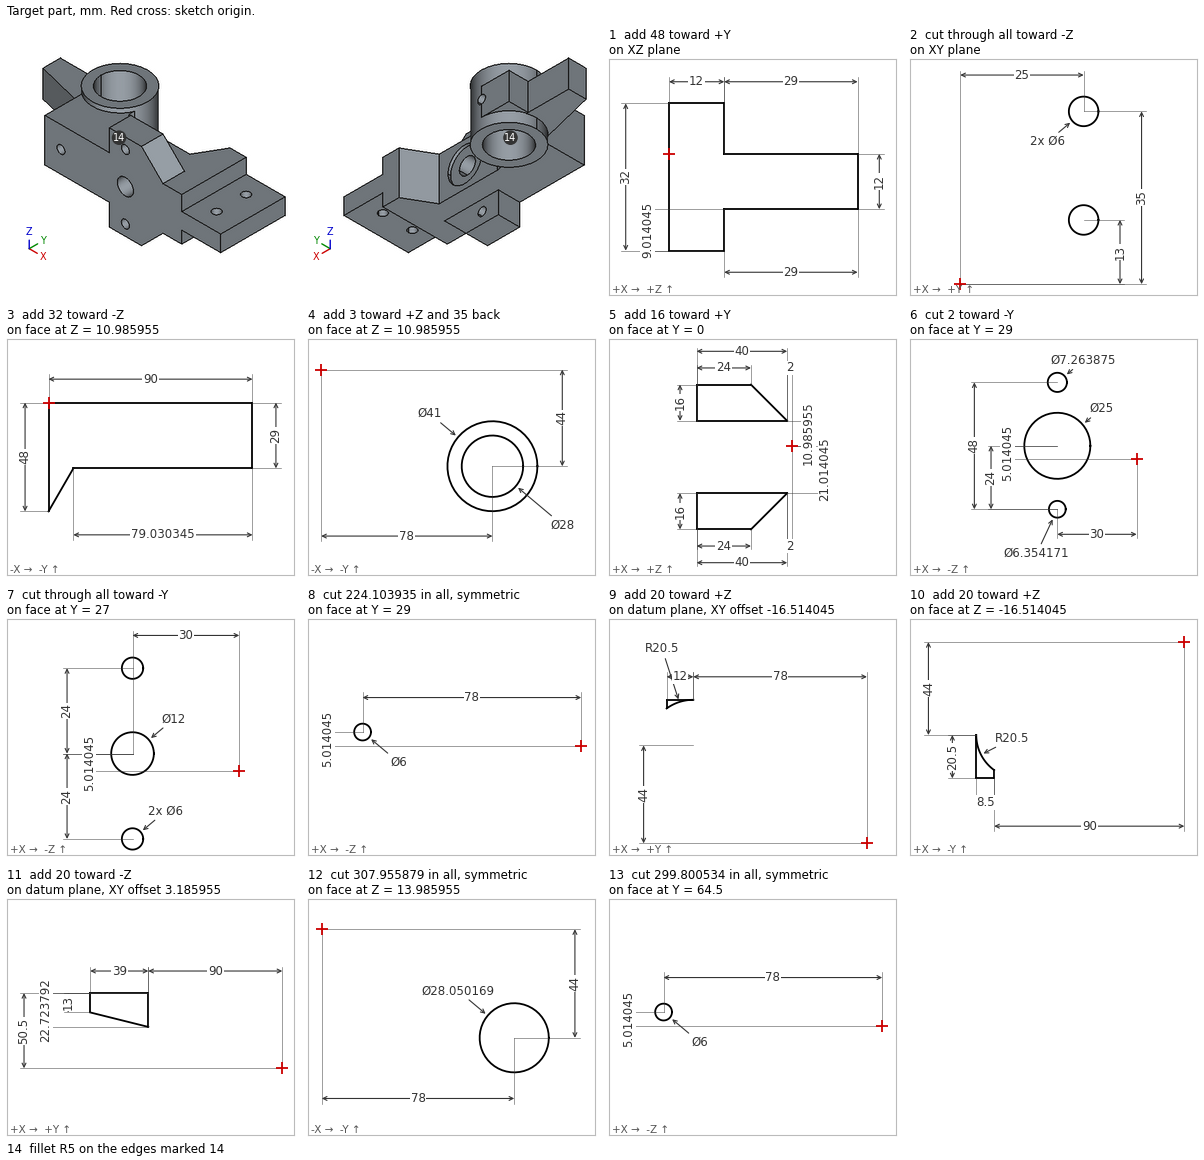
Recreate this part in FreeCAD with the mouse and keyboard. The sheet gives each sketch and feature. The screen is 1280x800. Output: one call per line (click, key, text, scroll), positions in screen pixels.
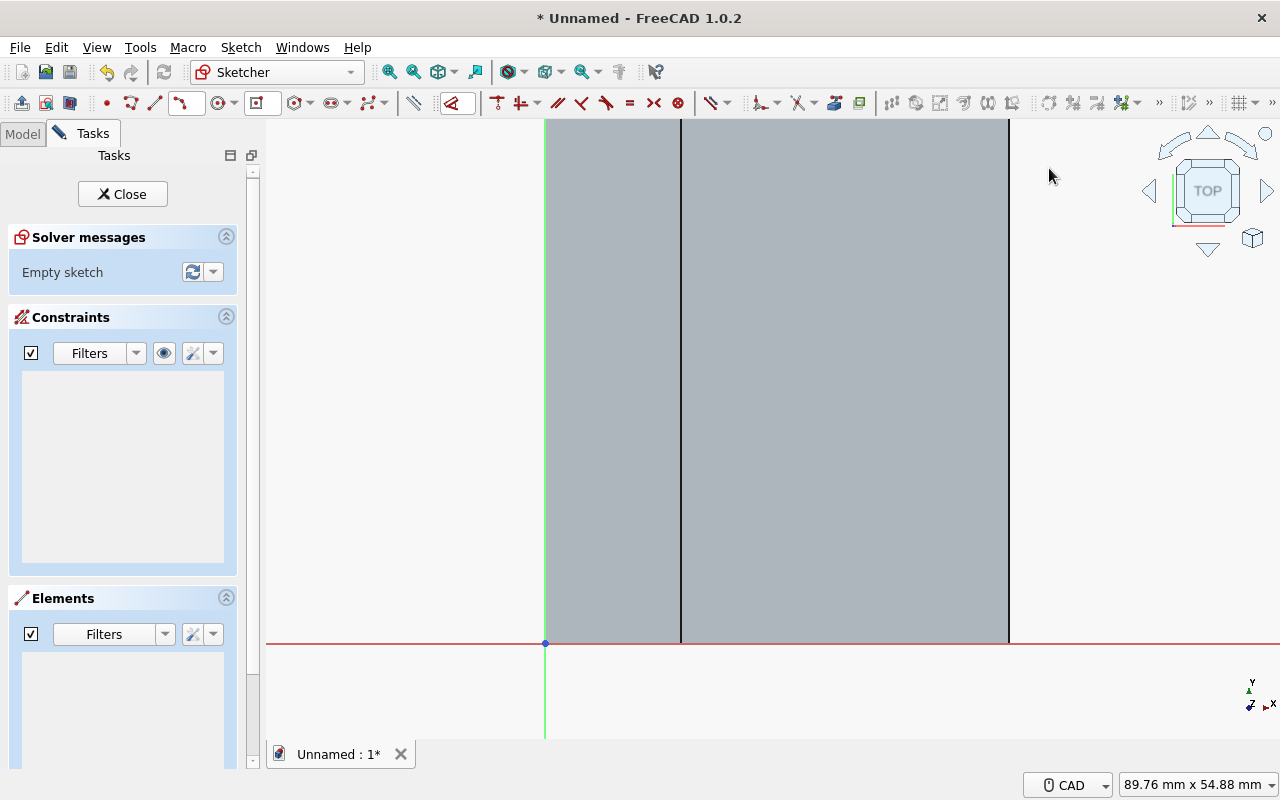
key(g)
key(c)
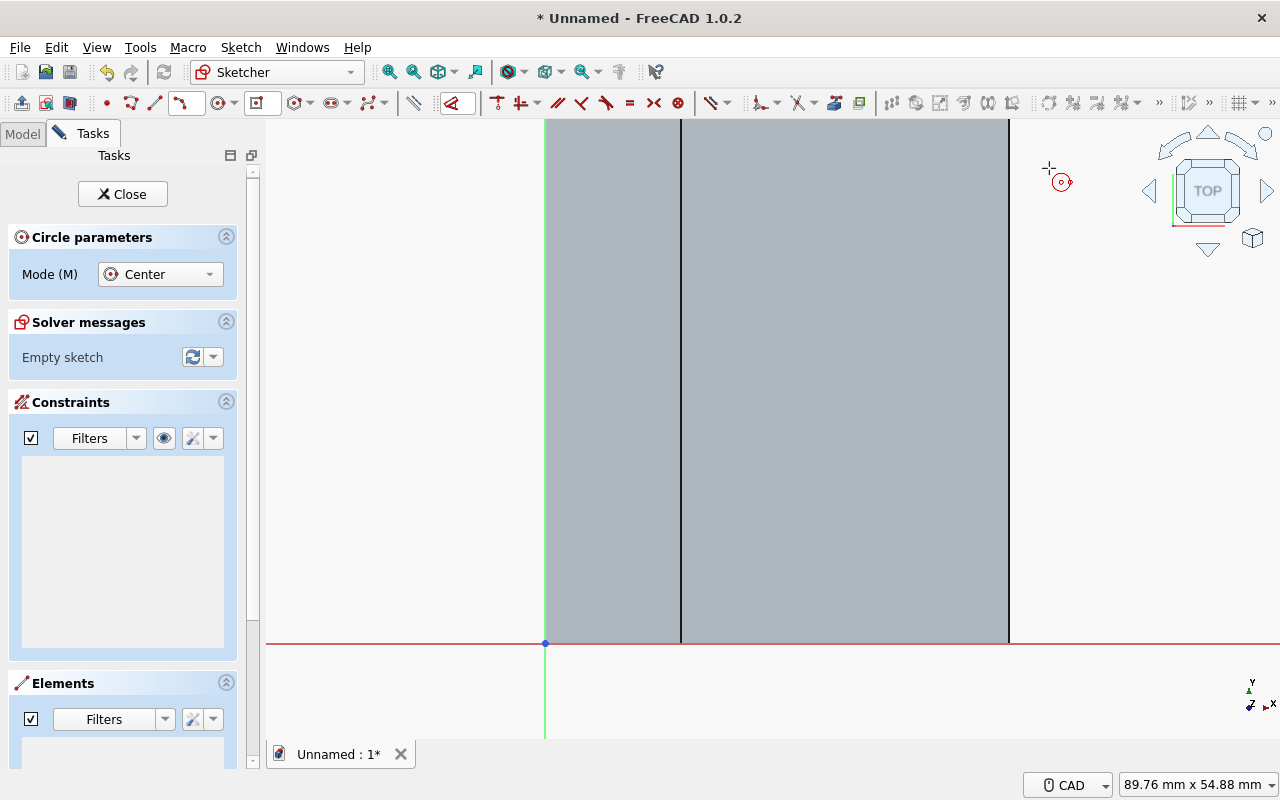
click(828, 248)
move(852, 224)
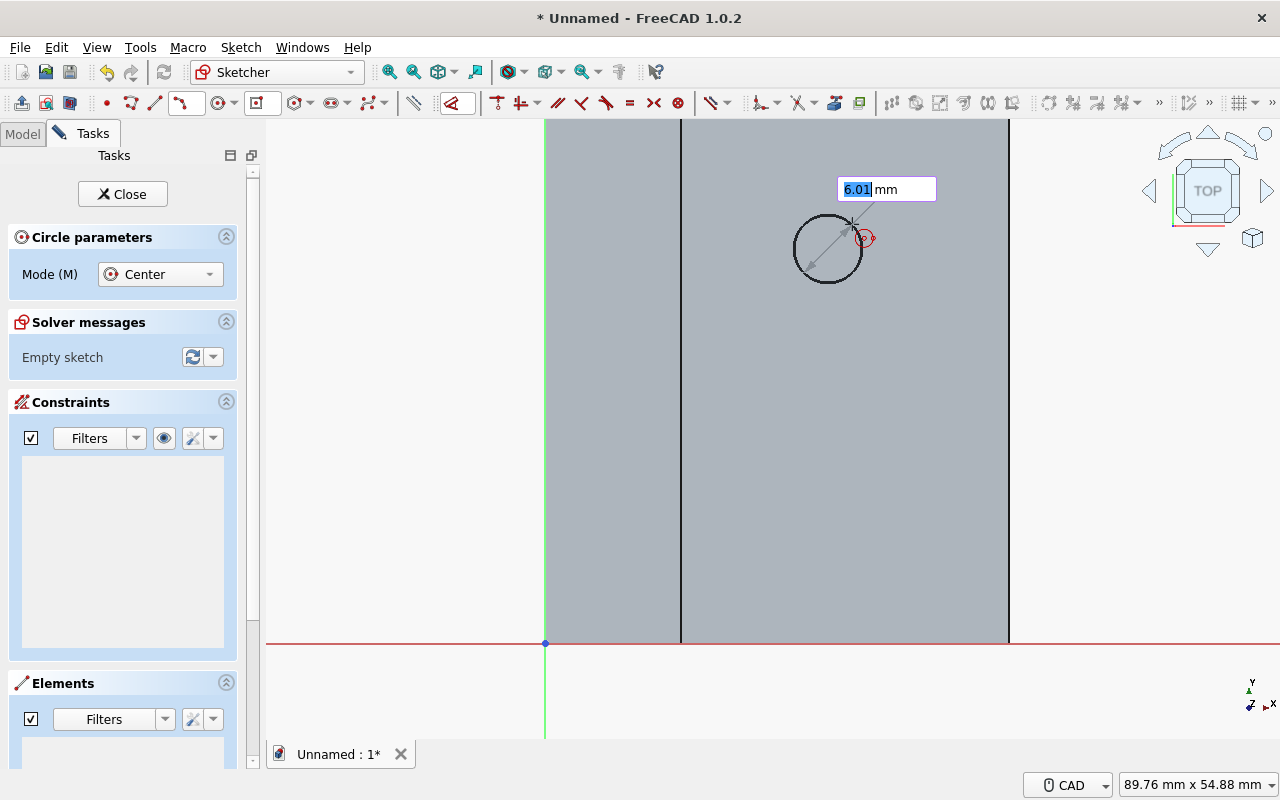
text(6)
key(Return)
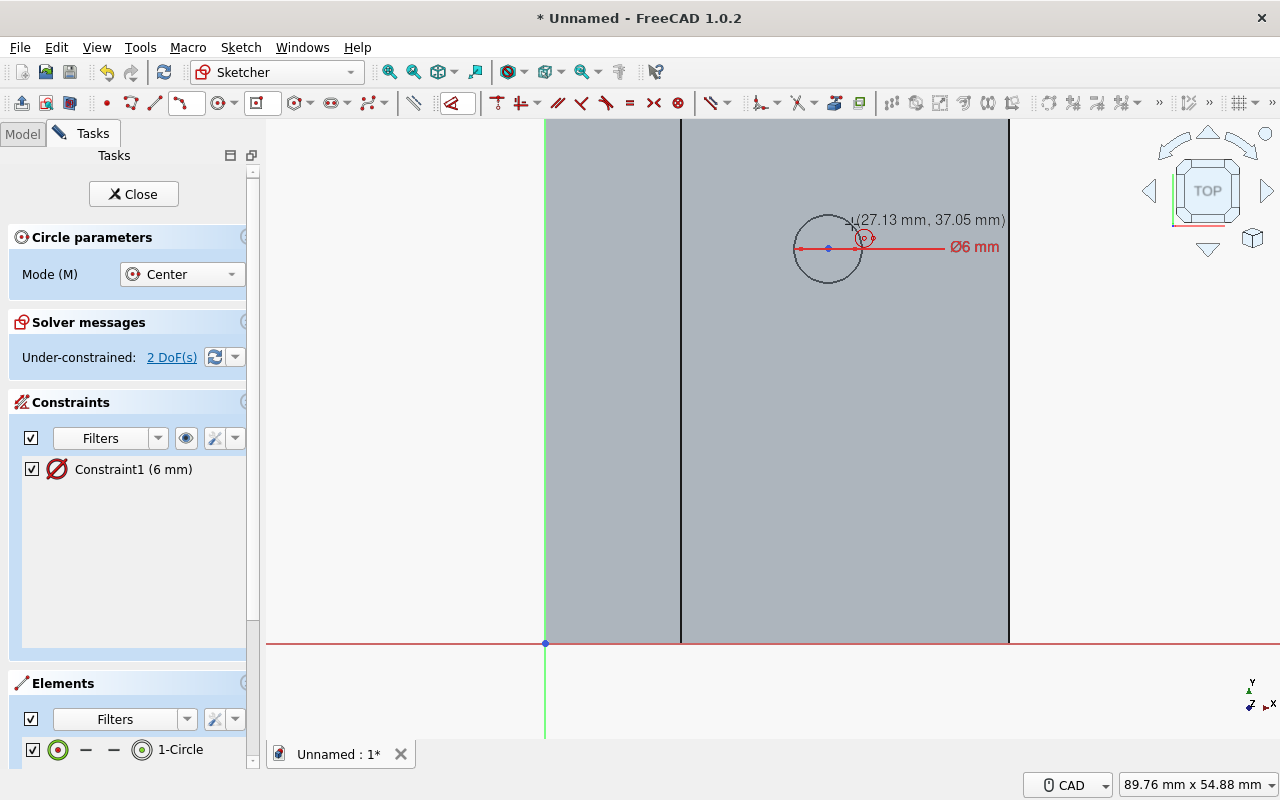
click(828, 497)
move(852, 473)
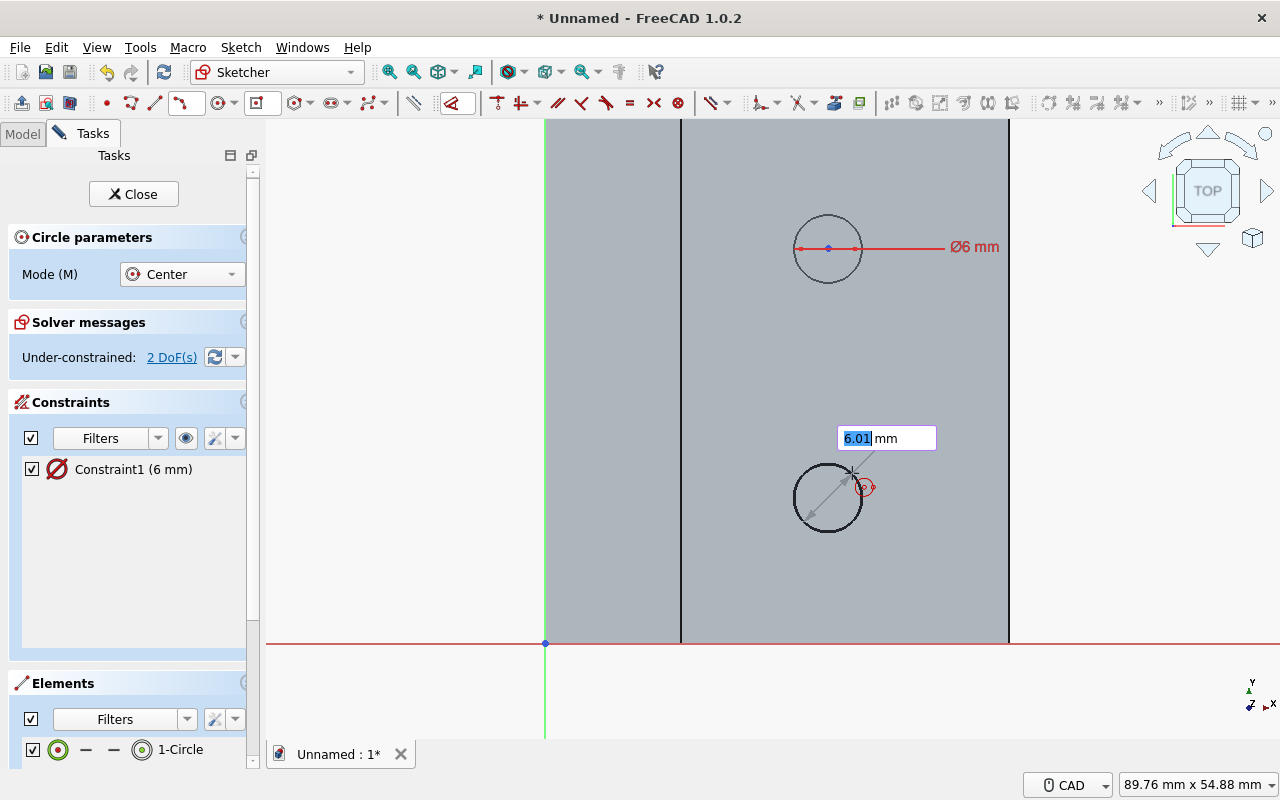
text(6)
key(Return)
key(Escape)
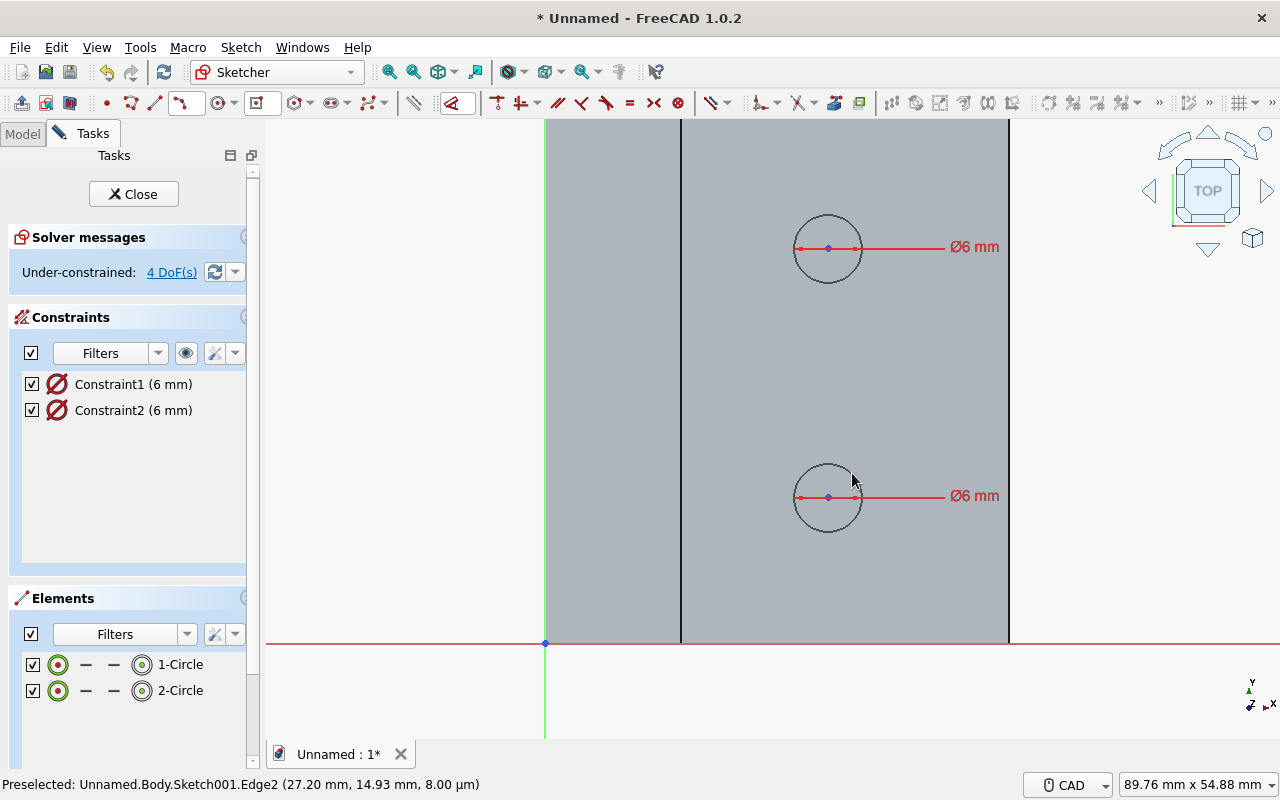
click(828, 249)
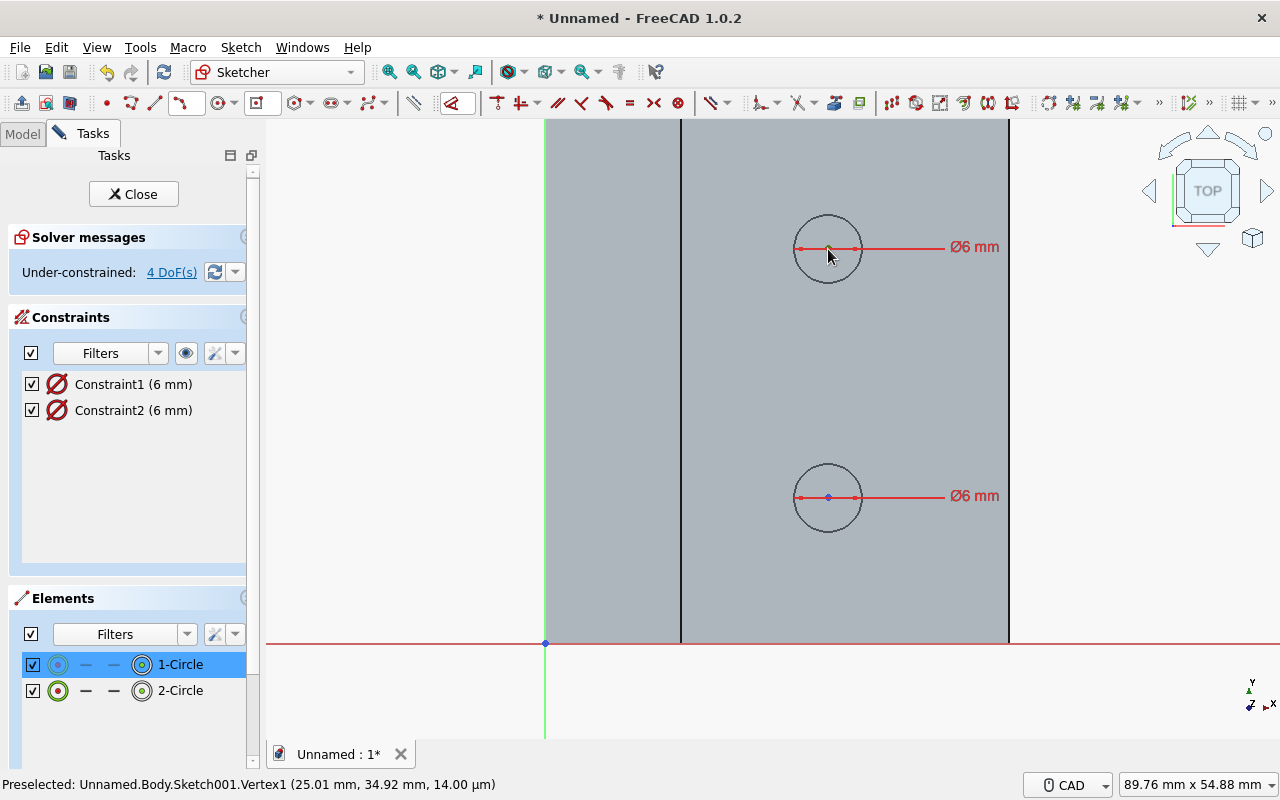
click(828, 498)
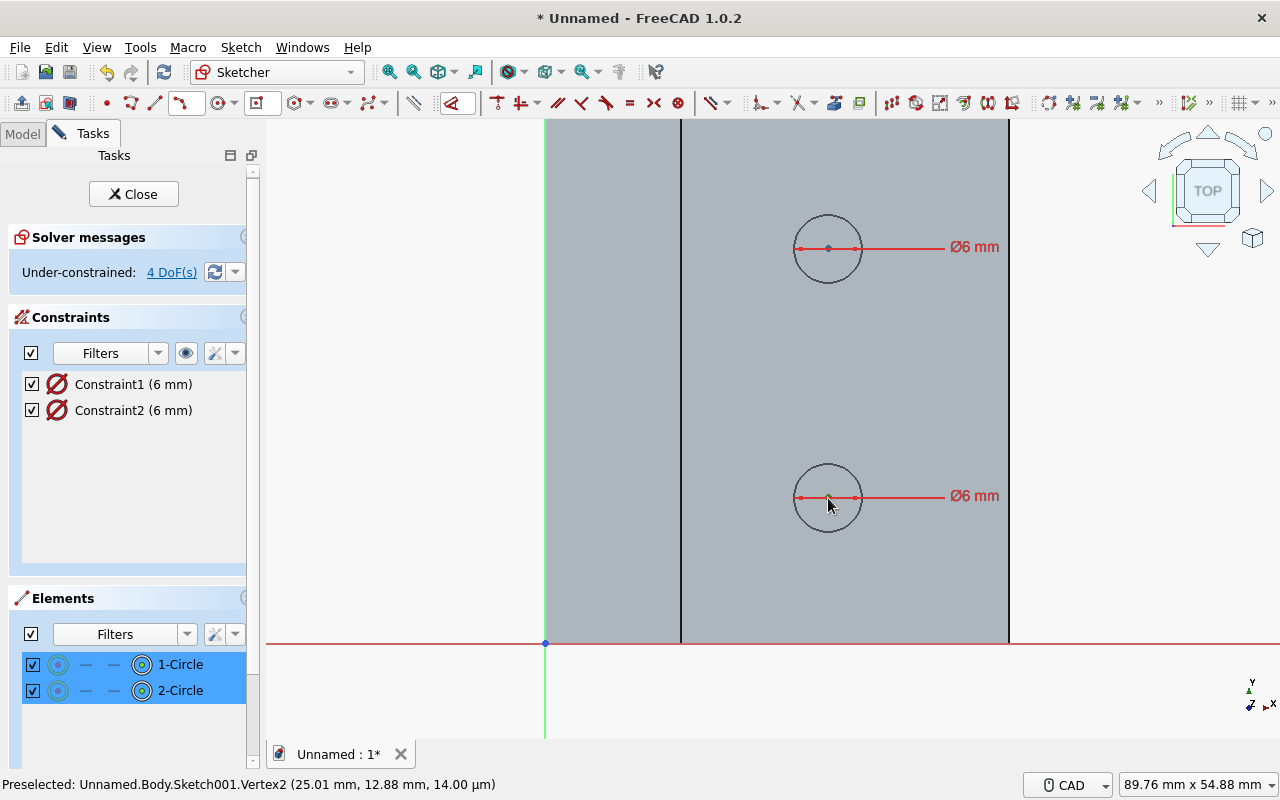
click(540, 104)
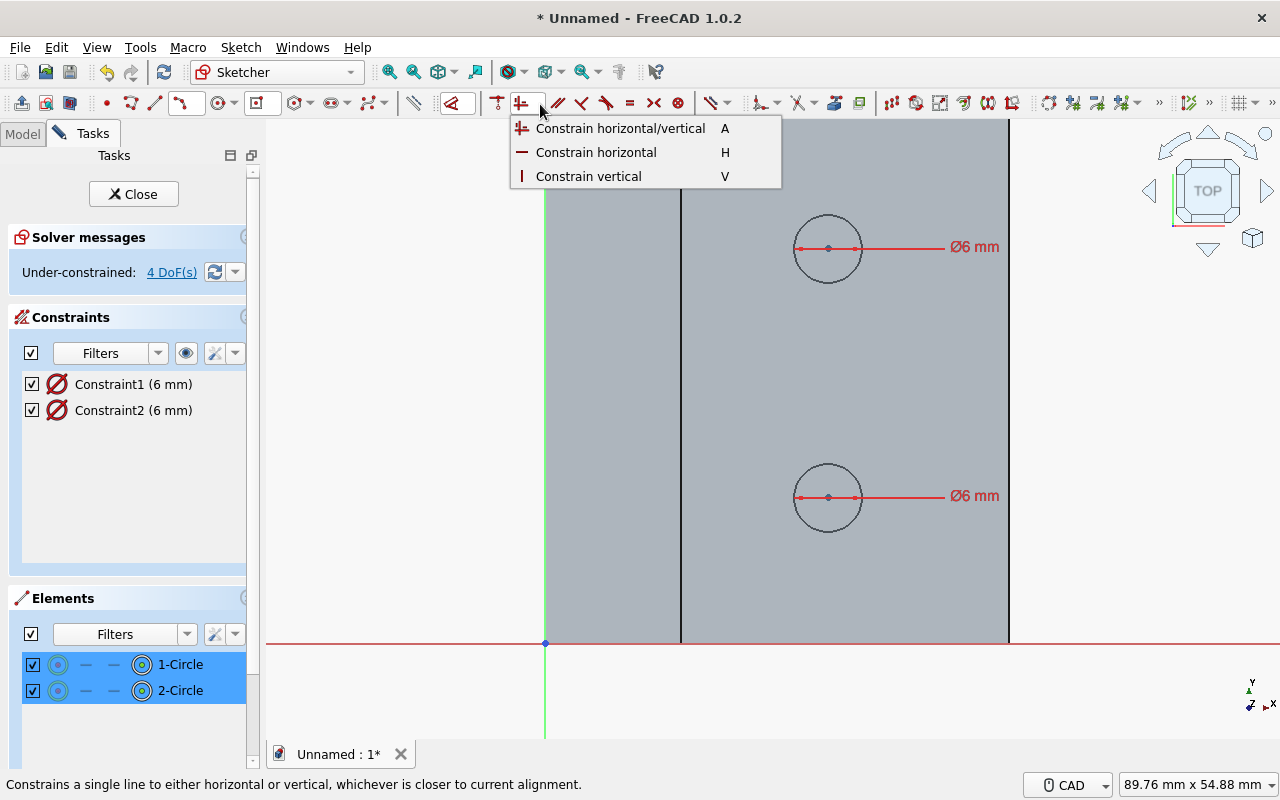
click(646, 176)